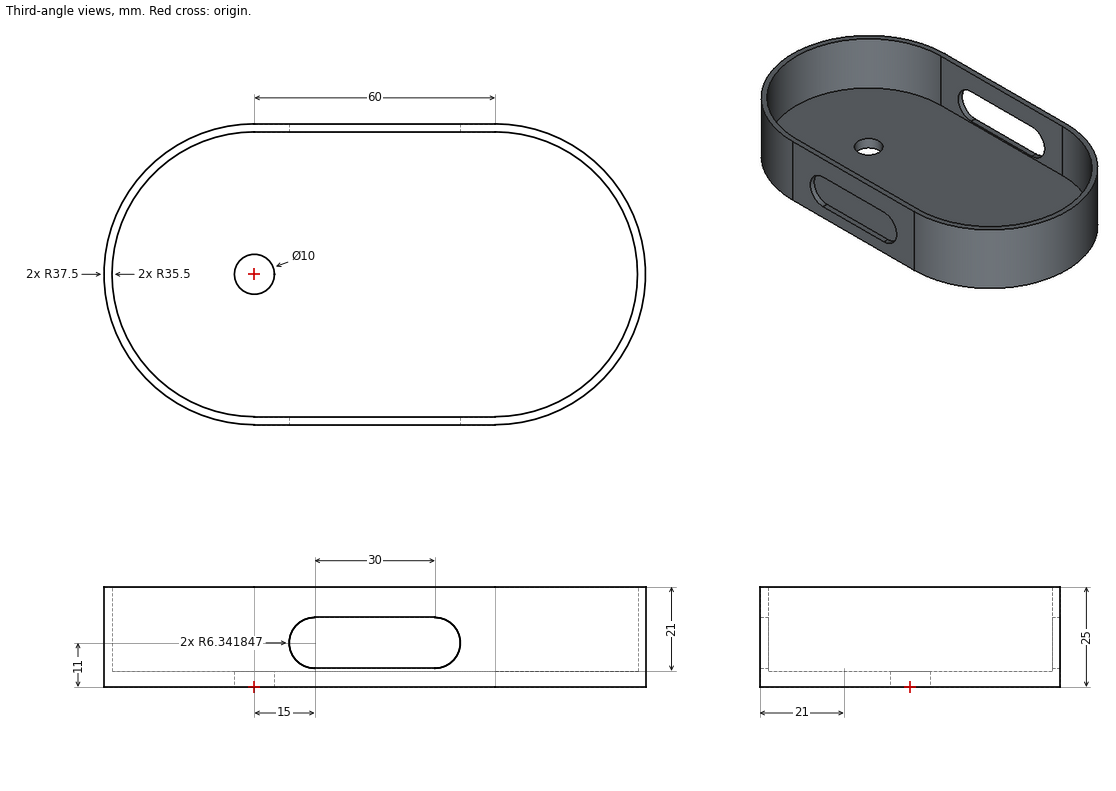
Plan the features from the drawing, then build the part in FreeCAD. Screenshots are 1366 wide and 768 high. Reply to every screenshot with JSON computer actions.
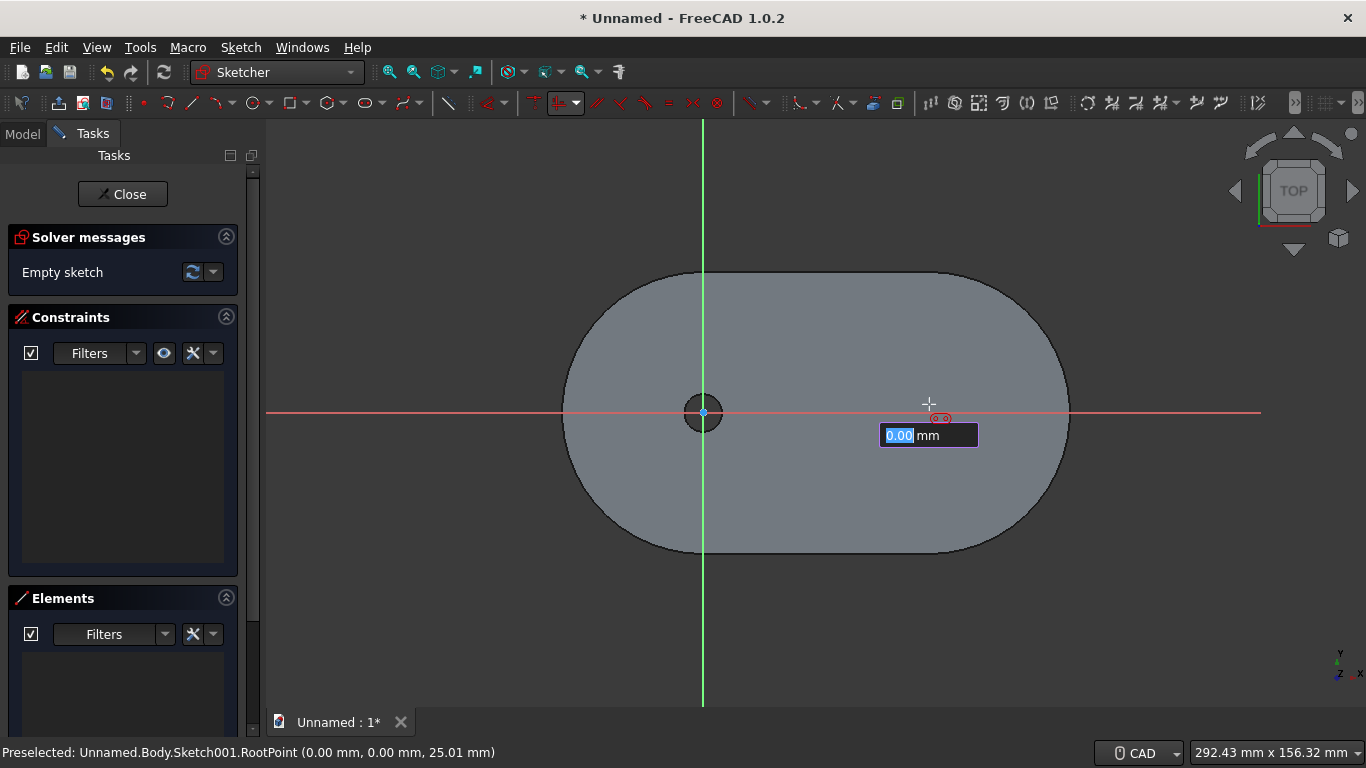
{"action": "left_click", "coordinate": [816, 279]}
{"action": "key", "text": "Escape"}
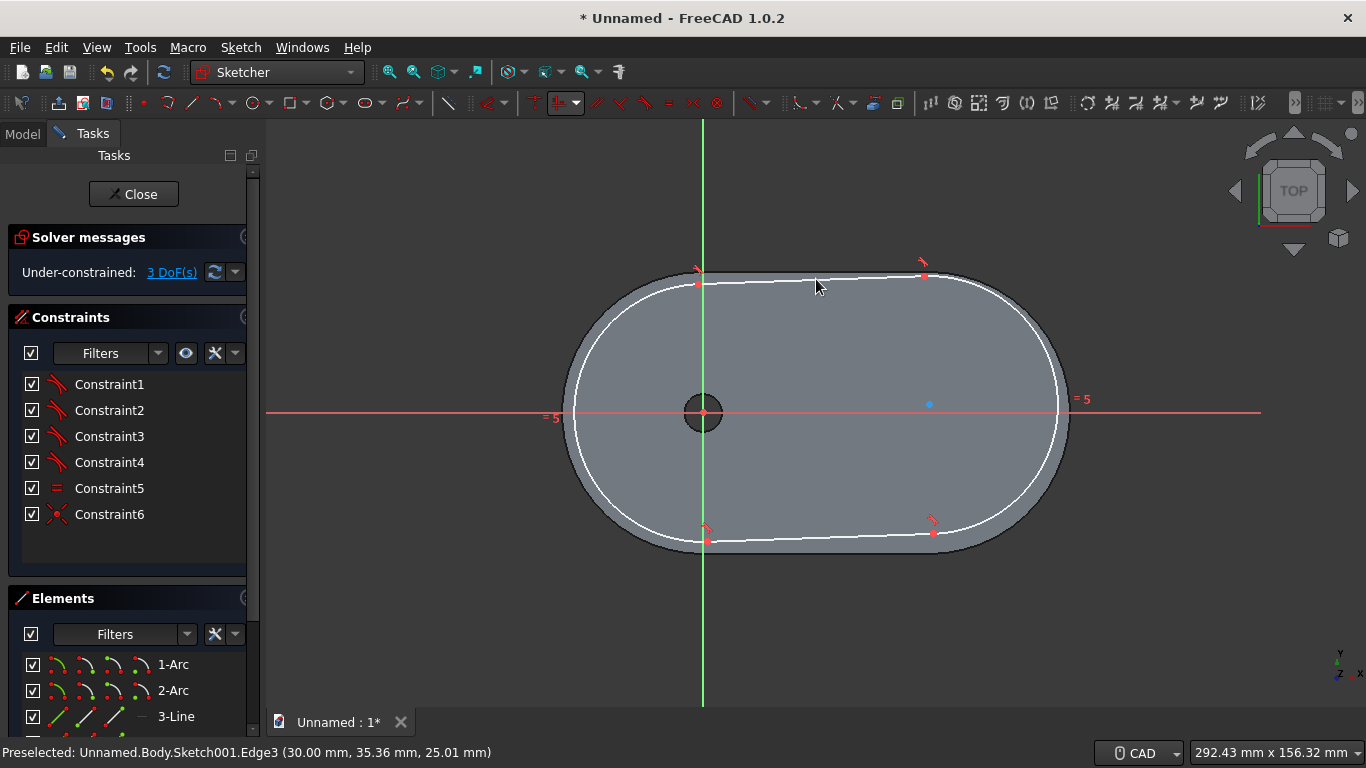
{"action": "left_click", "coordinate": [766, 282]}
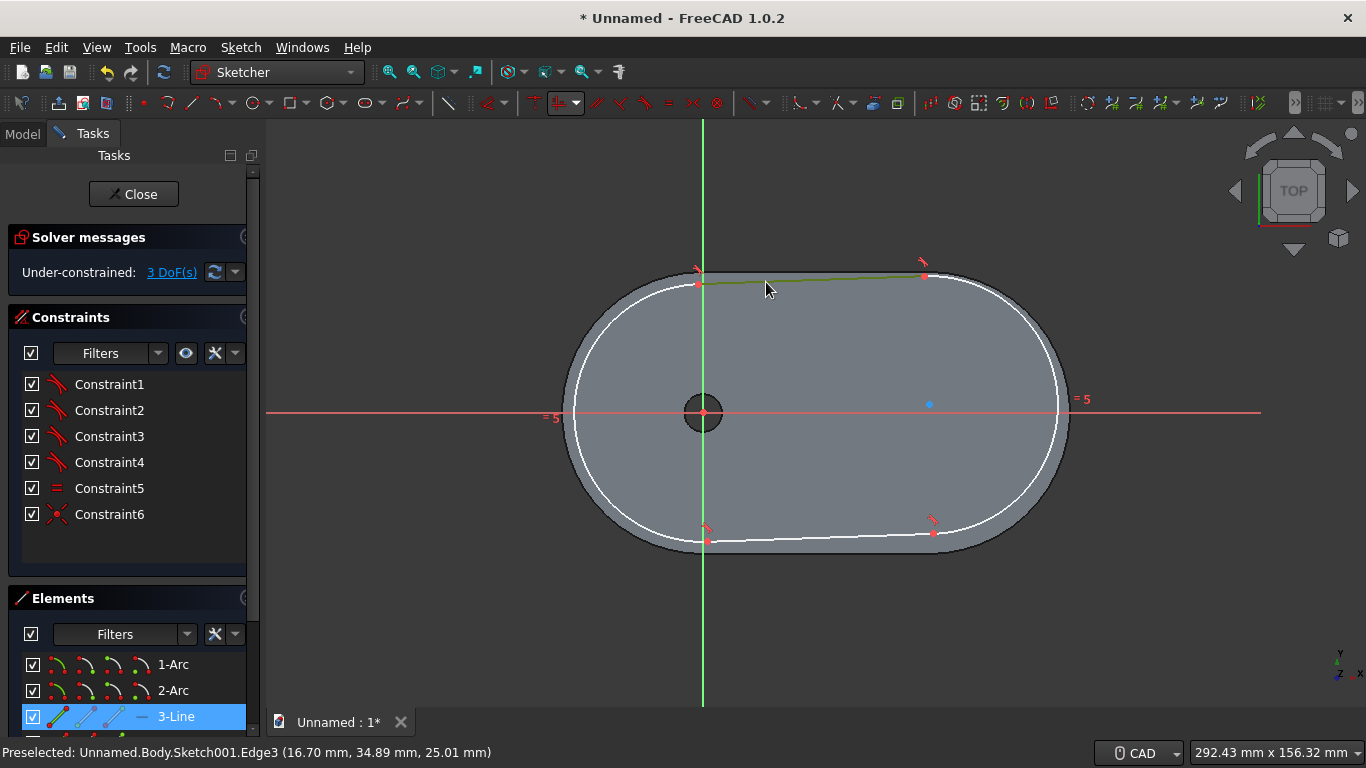
{"action": "left_click", "coordinate": [578, 104]}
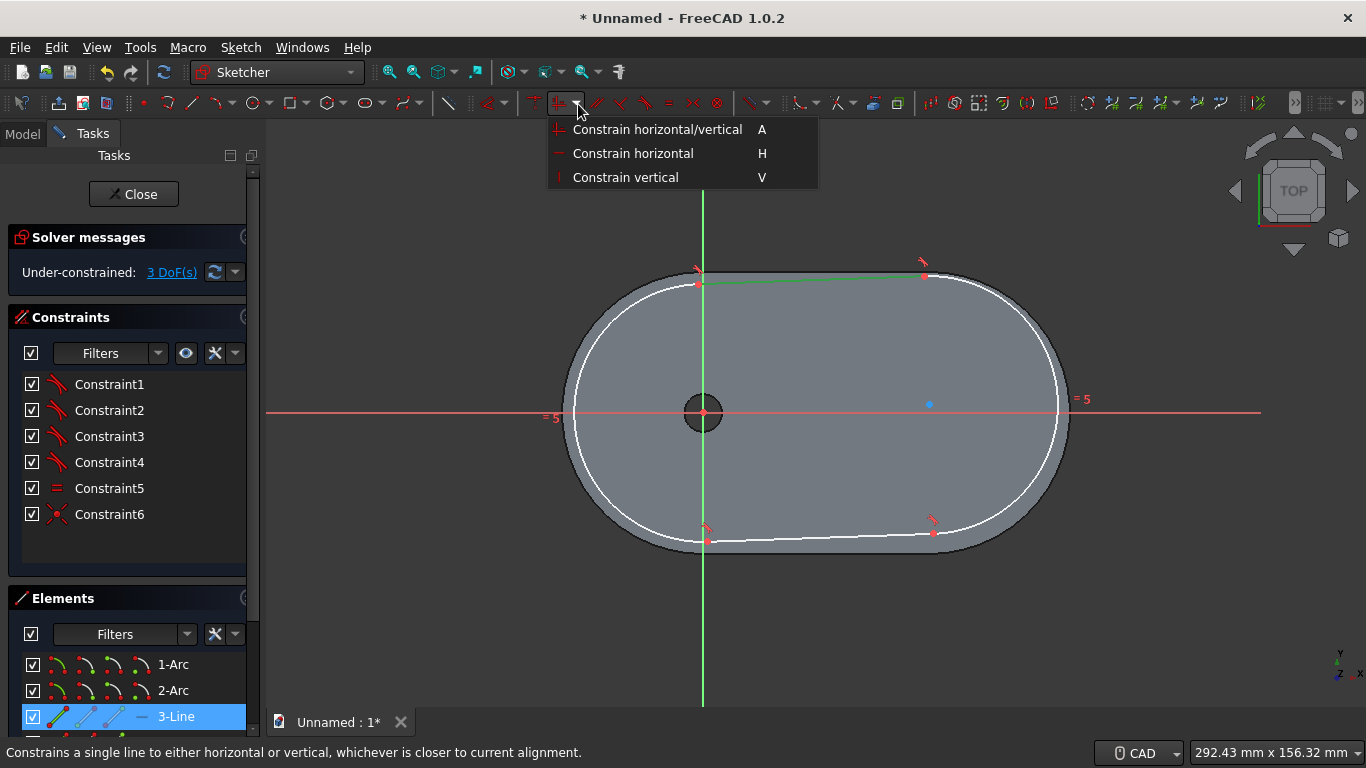
{"action": "left_click", "coordinate": [683, 153]}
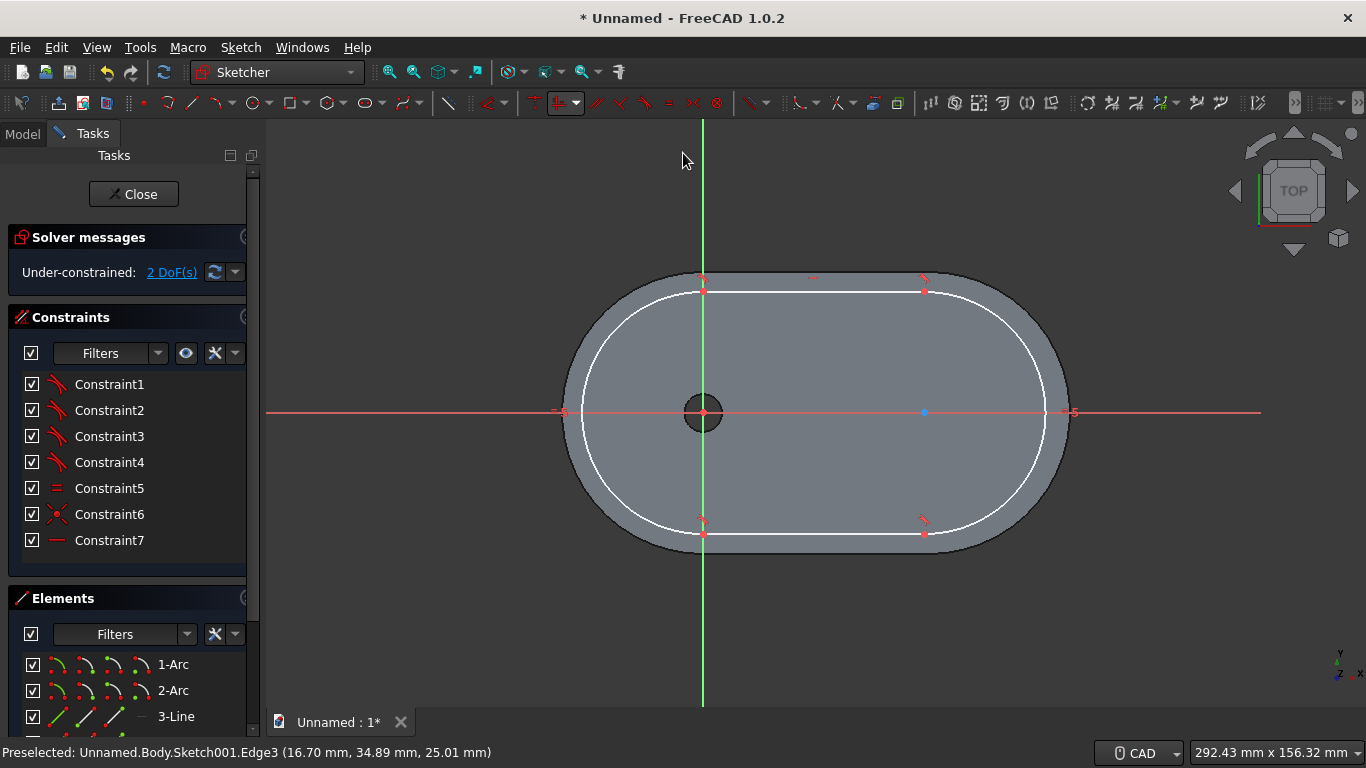
{"action": "left_click", "coordinate": [488, 104]}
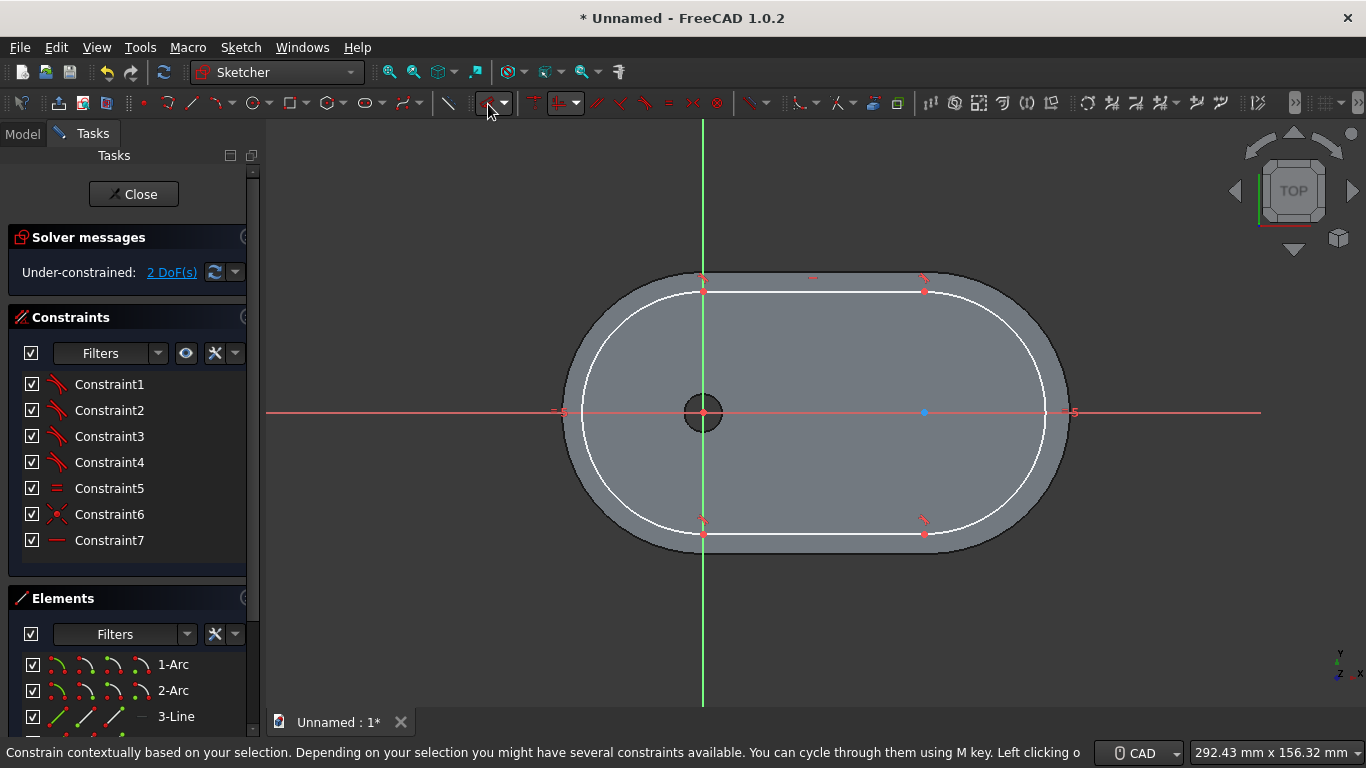
{"action": "left_click", "coordinate": [605, 342]}
{"action": "left_click", "coordinate": [579, 323]}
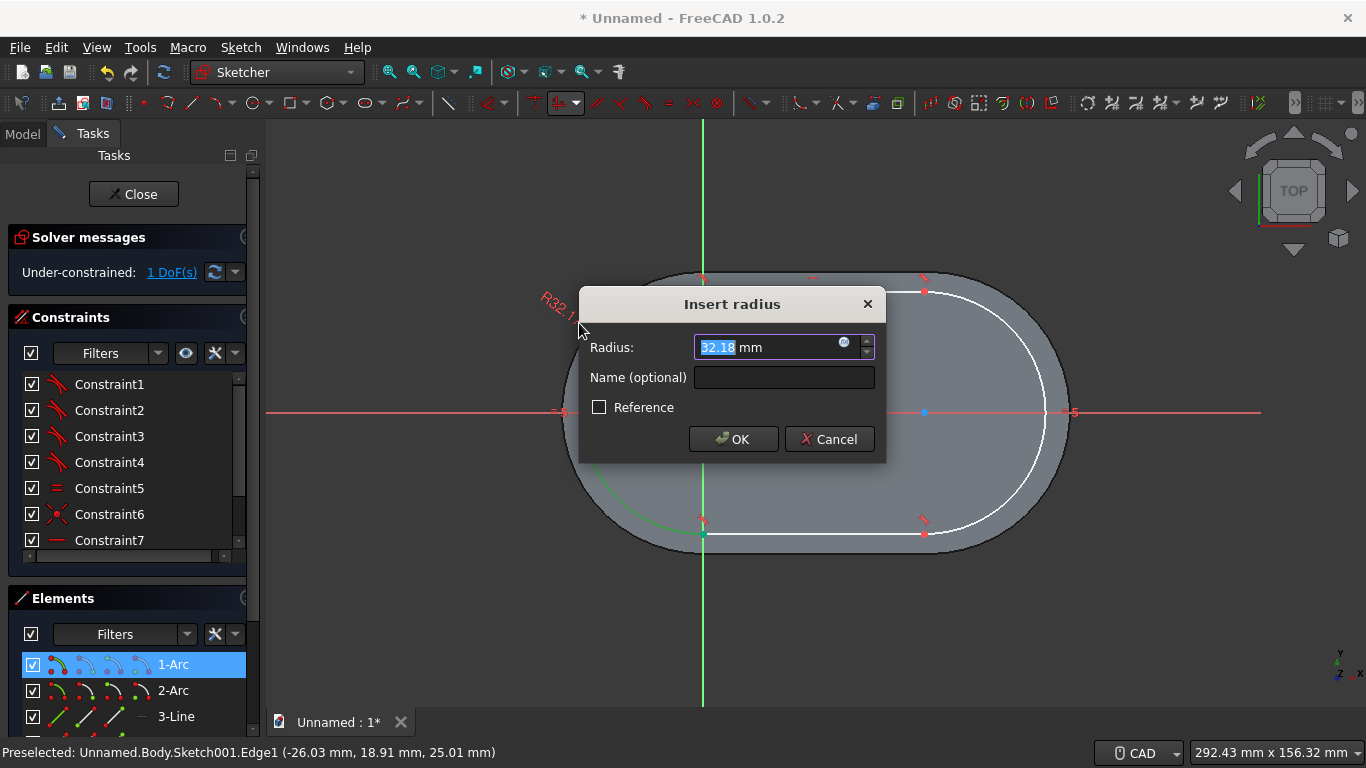
{"action": "type", "text": "35.5"}
{"action": "key", "text": "Return"}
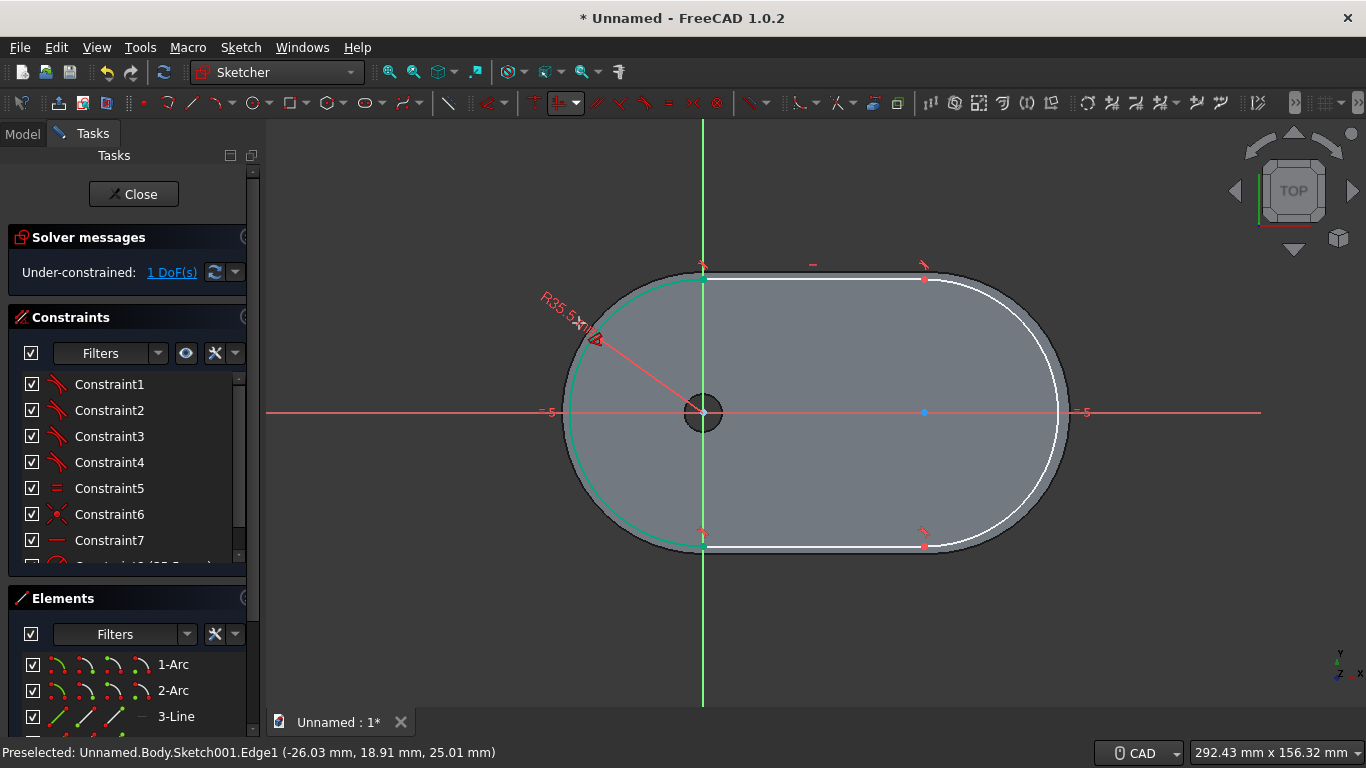
{"action": "left_click", "coordinate": [770, 279]}
{"action": "left_click", "coordinate": [814, 245]}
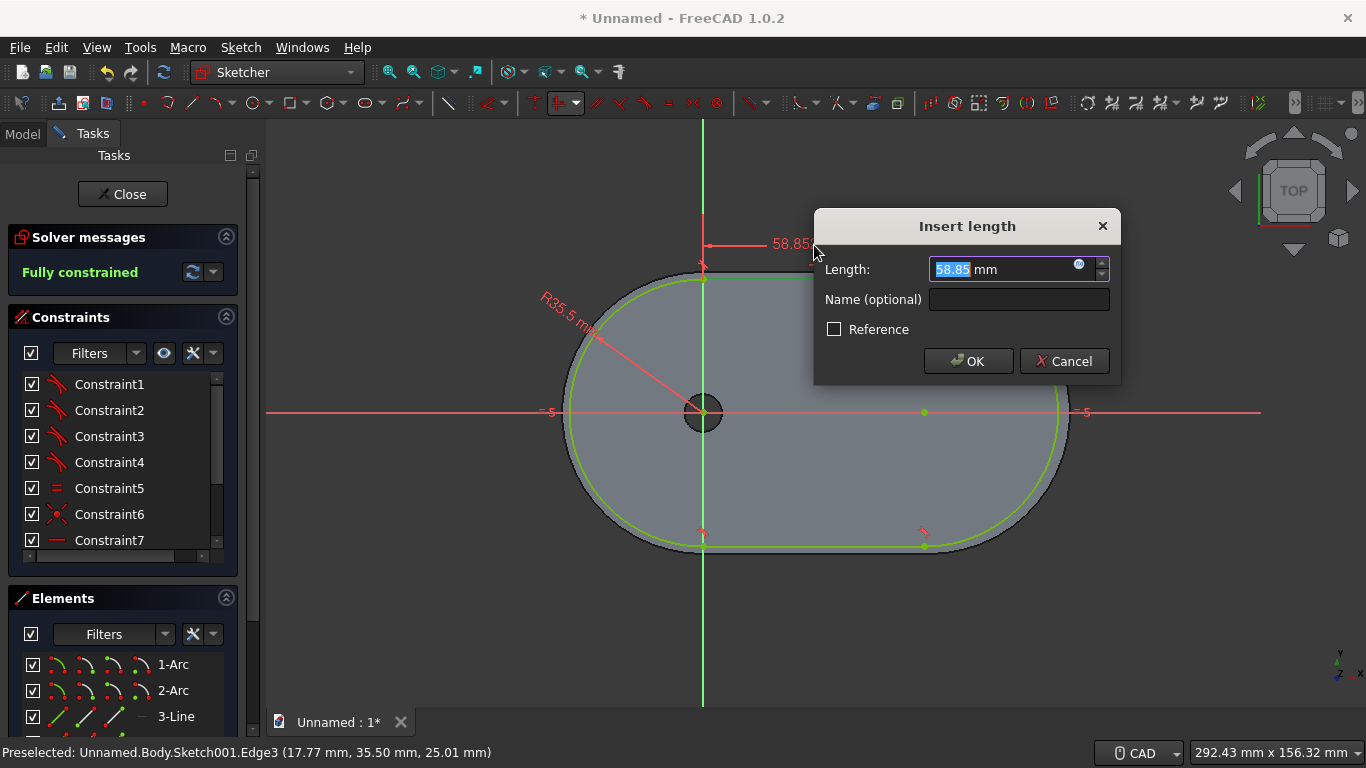
{"action": "type", "text": "60"}
{"action": "key", "text": "Return"}
{"action": "key", "text": "Escape"}